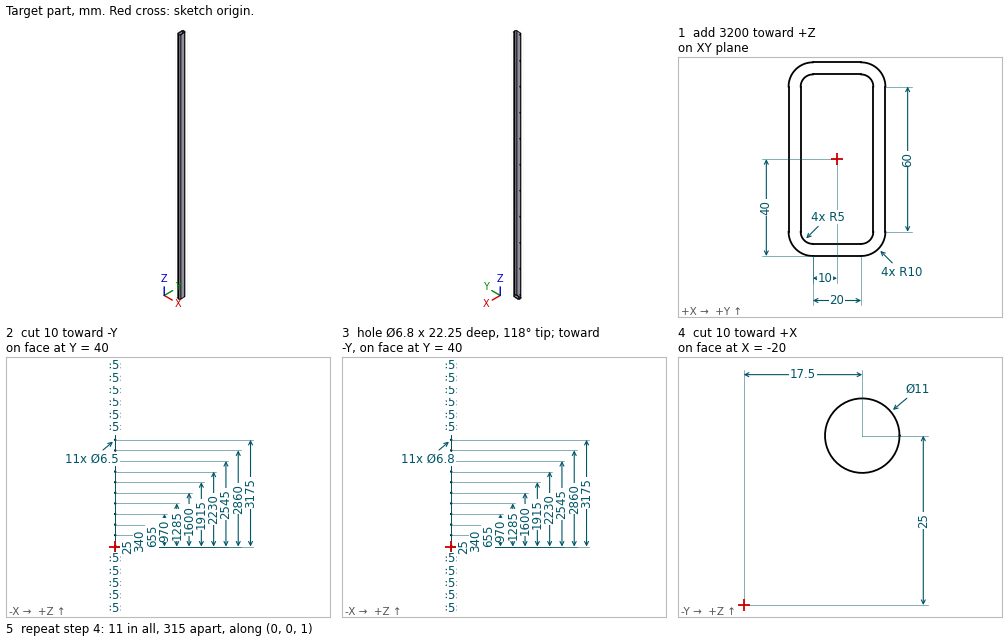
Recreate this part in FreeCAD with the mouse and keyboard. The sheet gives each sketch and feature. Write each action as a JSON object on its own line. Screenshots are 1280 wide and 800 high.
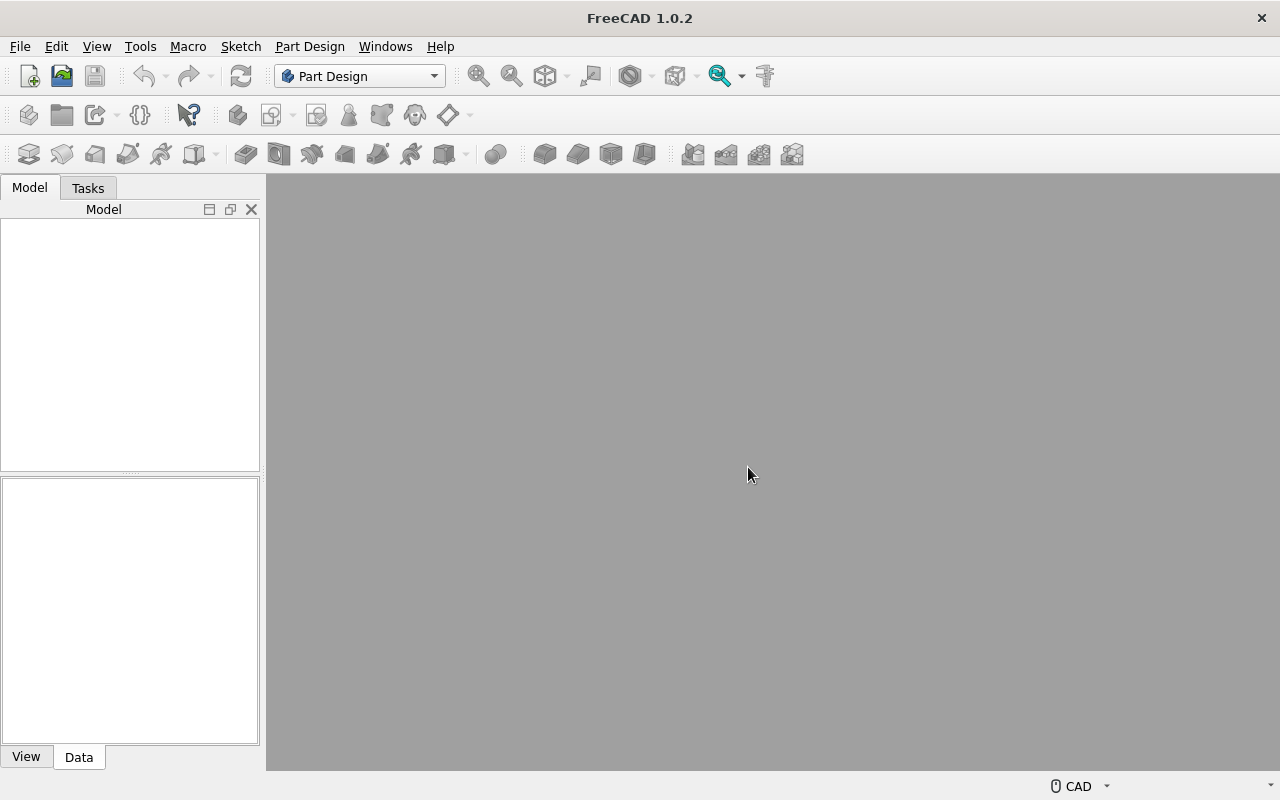
{"action": "left_click", "coordinate": [29, 76]}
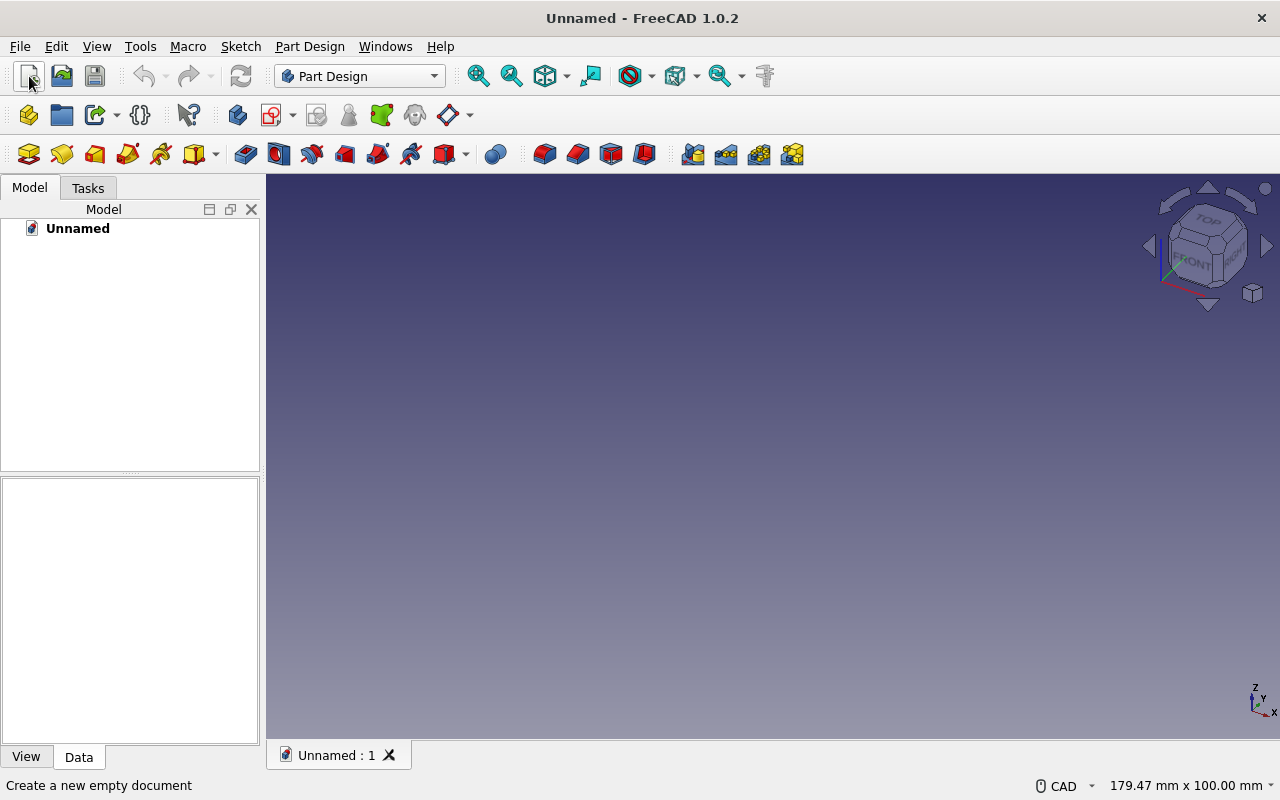
{"action": "left_click", "coordinate": [270, 116]}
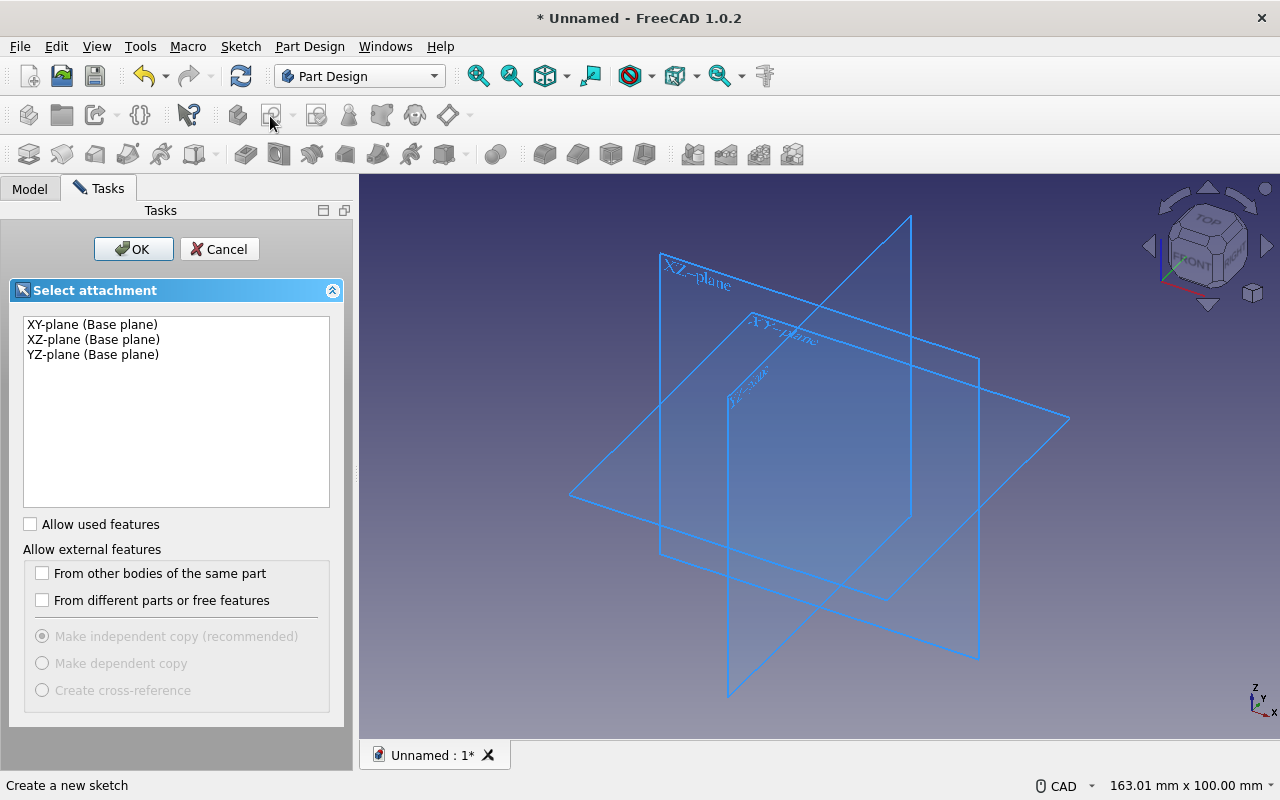
{"action": "left_click", "coordinate": [84, 324]}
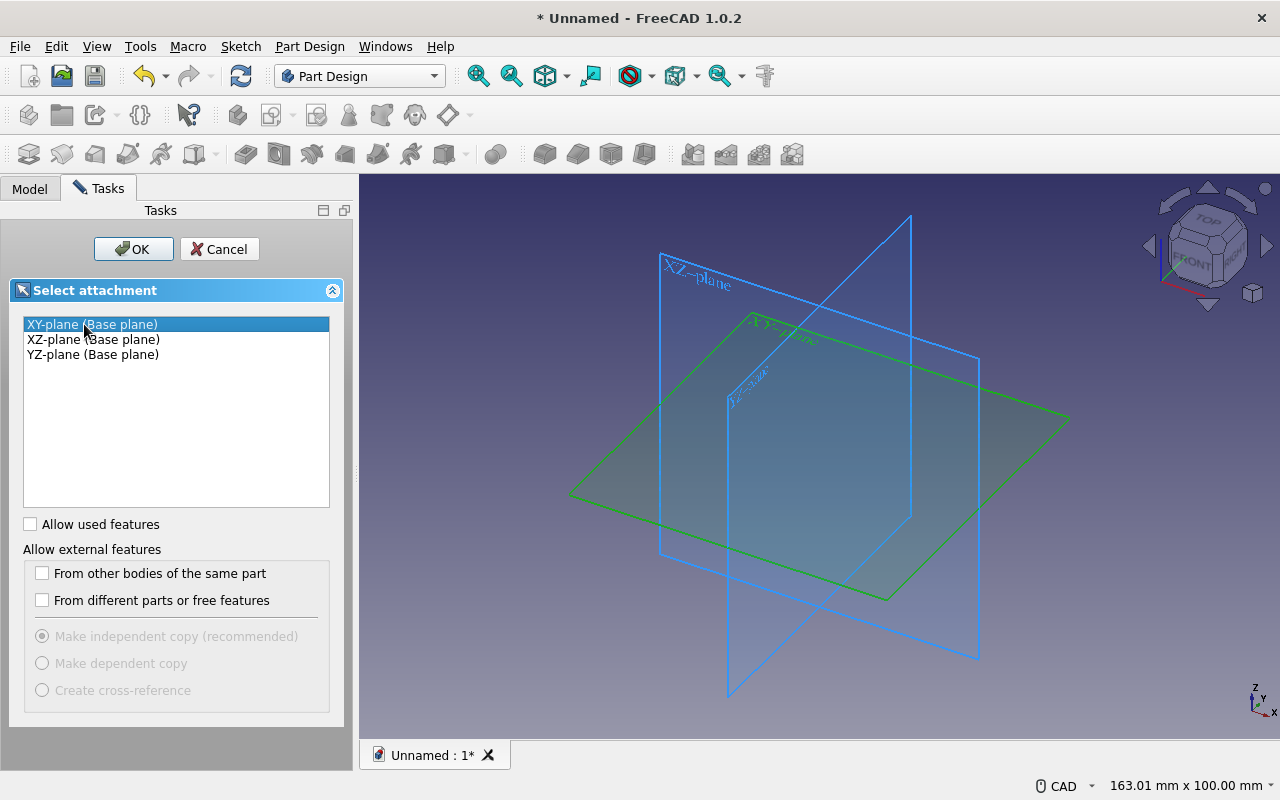
{"action": "left_click", "coordinate": [134, 249]}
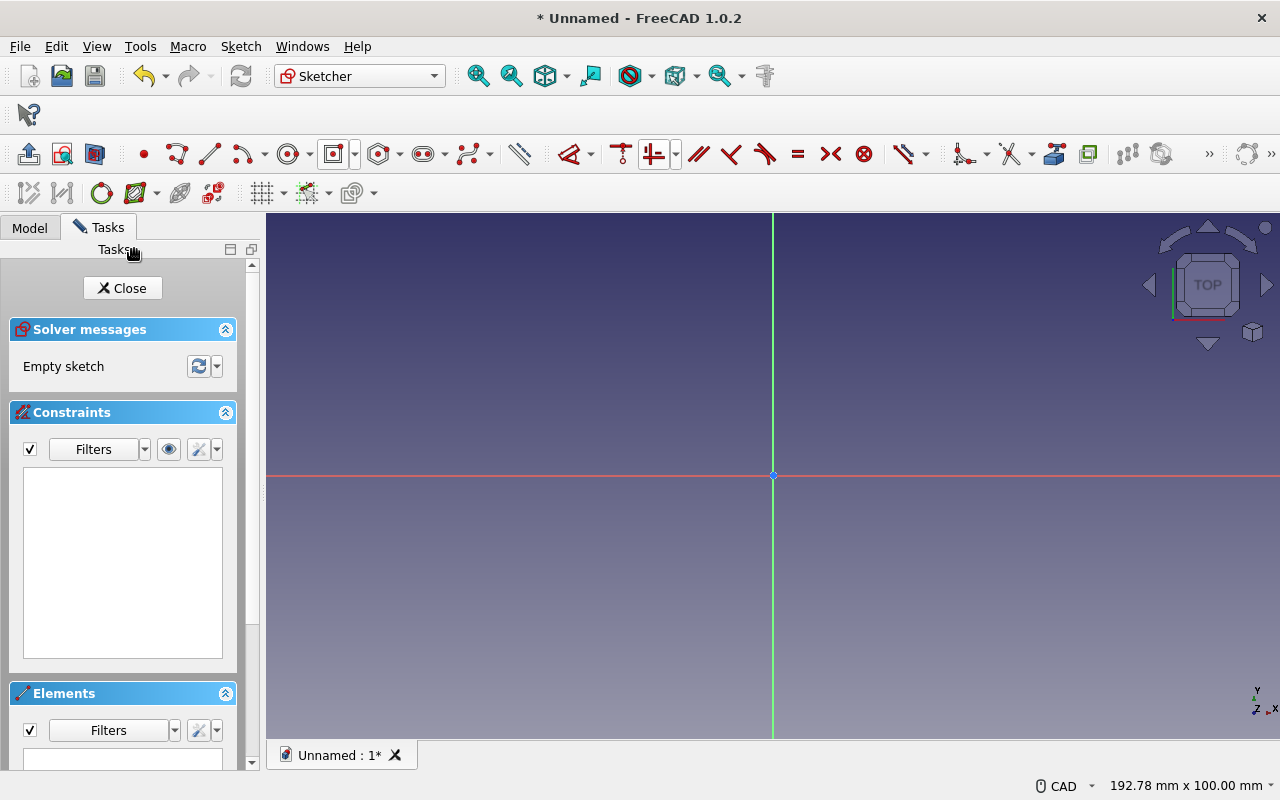
{"action": "scroll", "coordinate": [395, 476], "scroll_direction": "down", "scroll_amount": 1}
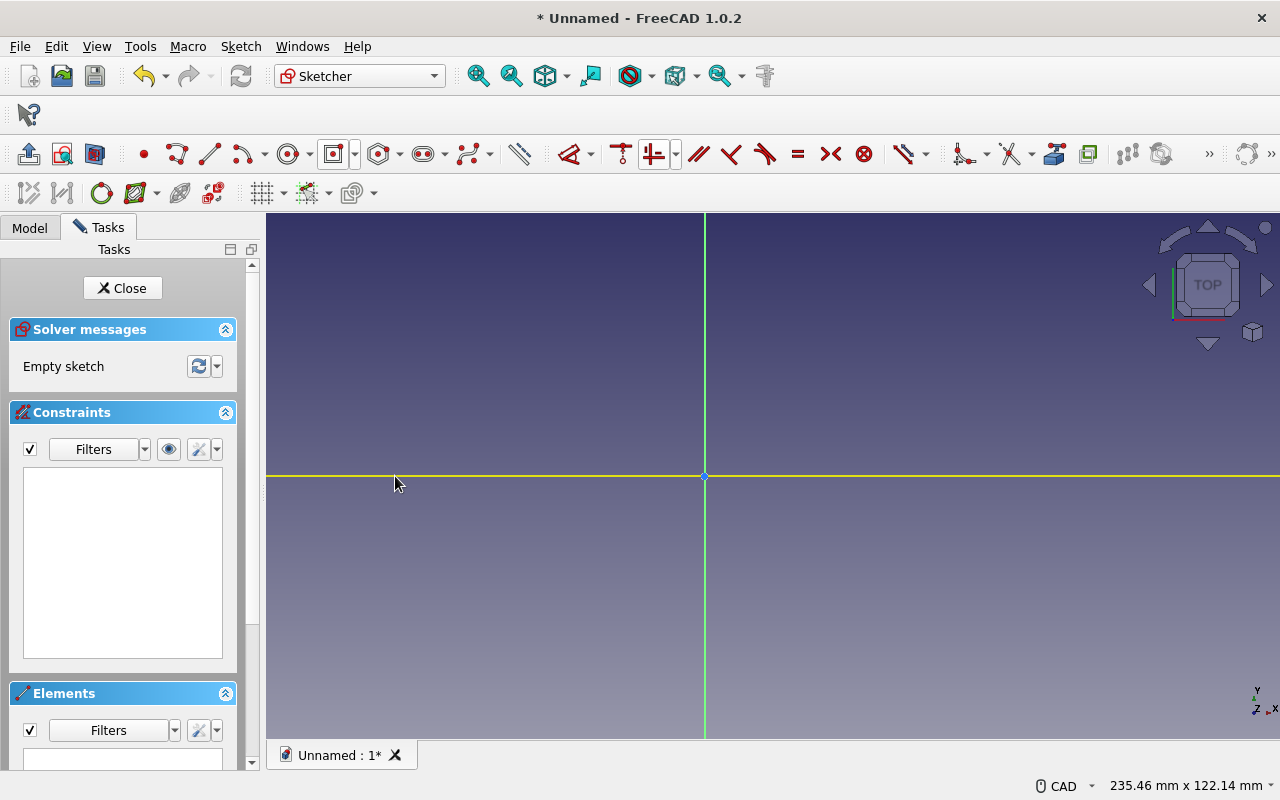
{"action": "left_click", "coordinate": [210, 154]}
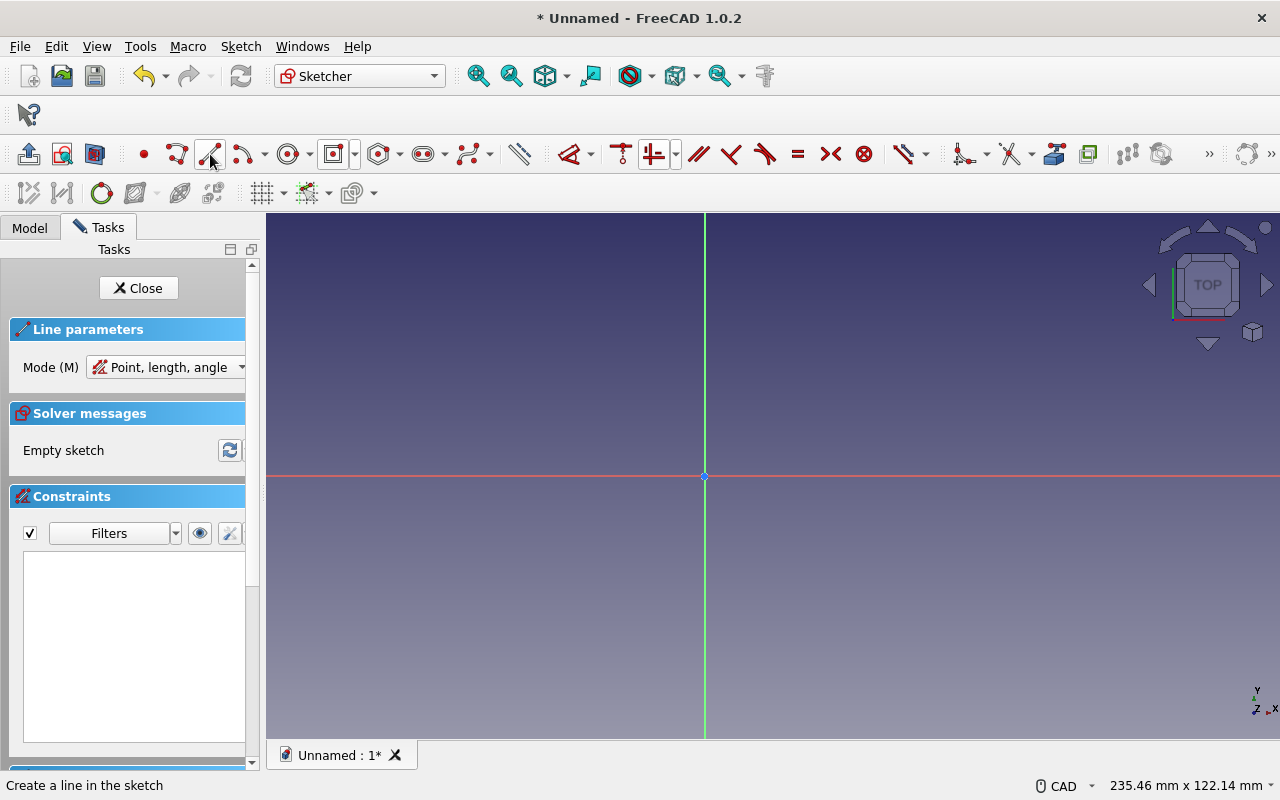
{"action": "left_click", "coordinate": [661, 648]}
{"action": "left_click", "coordinate": [748, 648]}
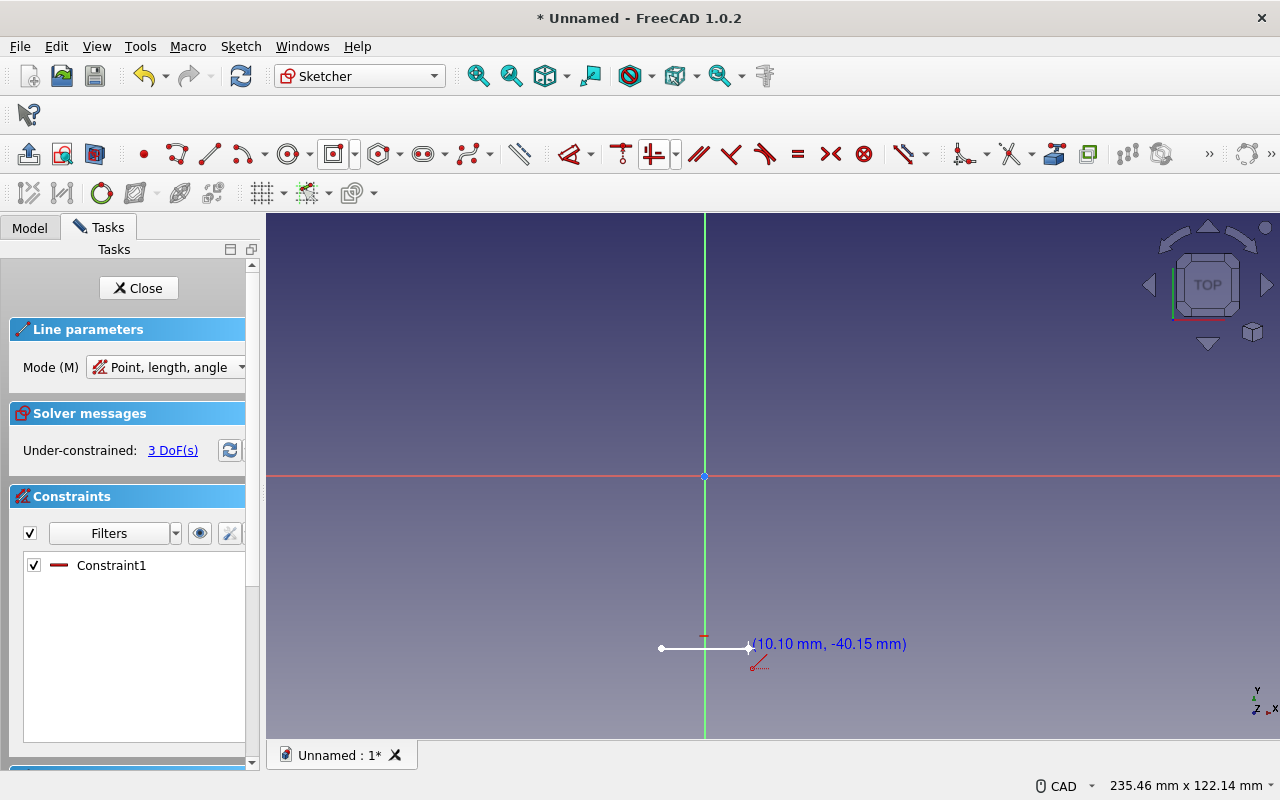
{"action": "left_click", "coordinate": [791, 605]}
{"action": "left_click", "coordinate": [791, 347]}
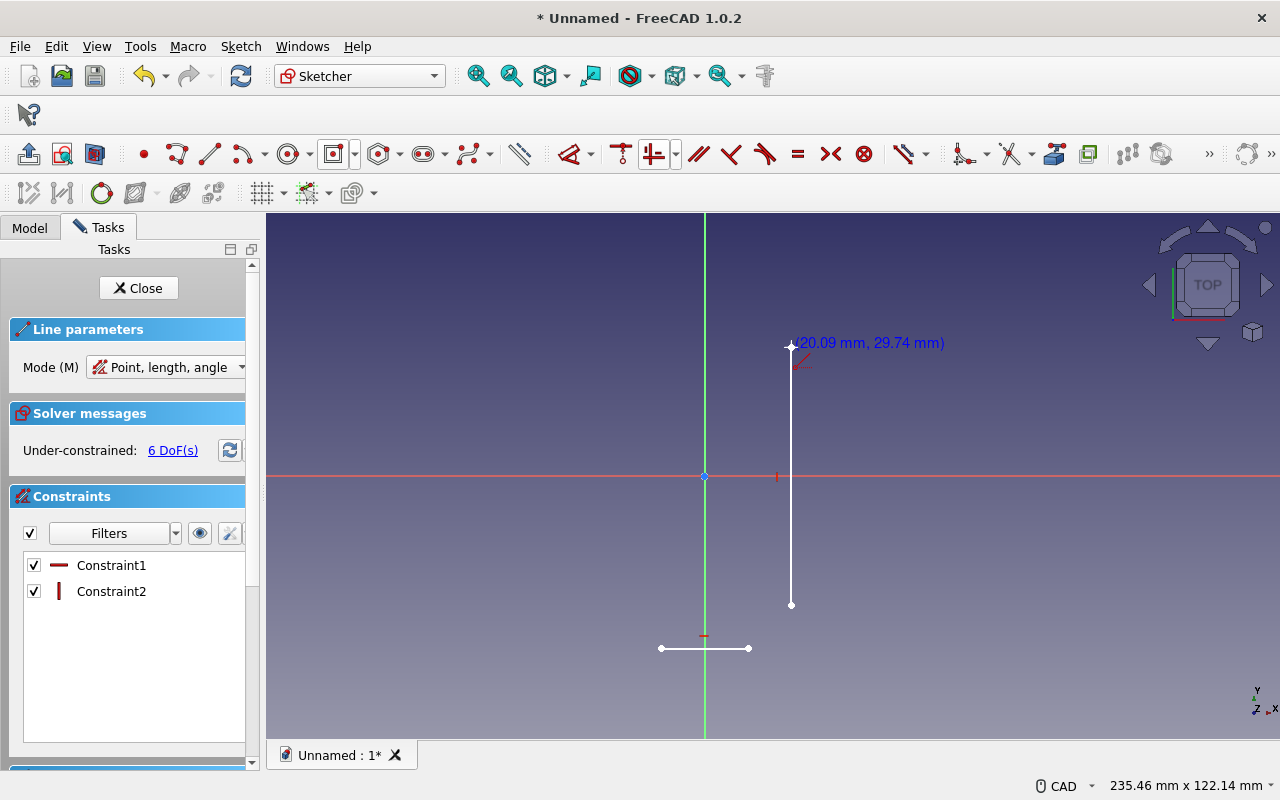
{"action": "left_click", "coordinate": [748, 304]}
{"action": "left_click", "coordinate": [661, 304]}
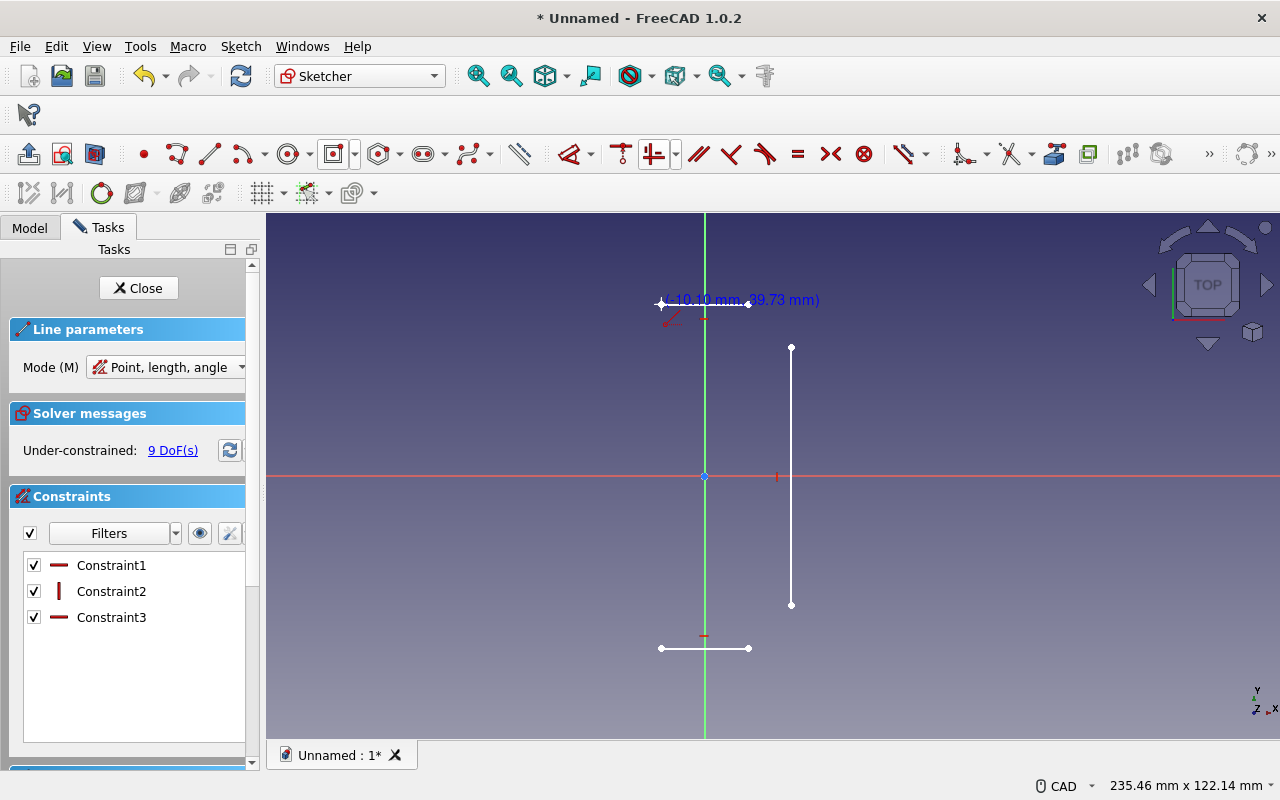
{"action": "left_click", "coordinate": [618, 347]}
{"action": "left_click", "coordinate": [618, 605]}